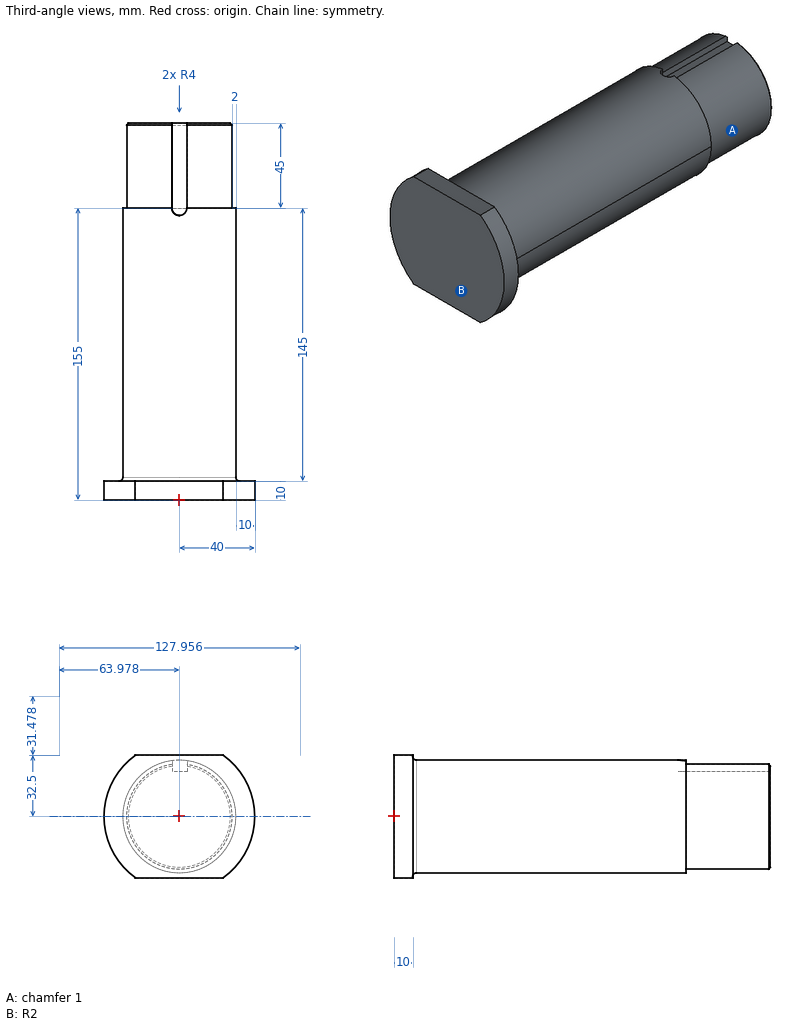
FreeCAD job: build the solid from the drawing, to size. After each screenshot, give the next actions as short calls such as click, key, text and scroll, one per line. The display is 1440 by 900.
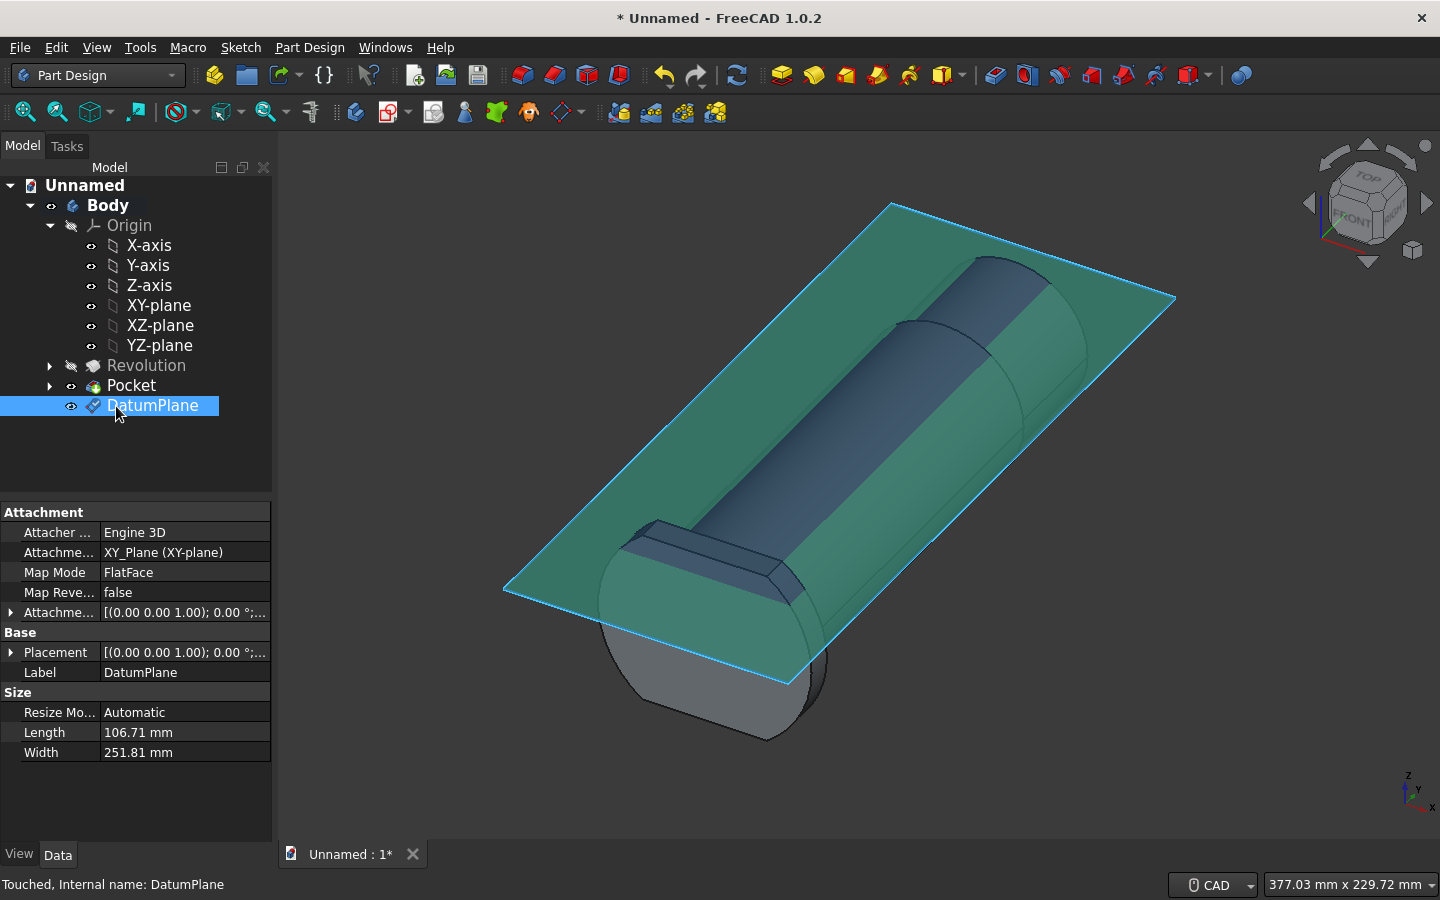
click(388, 112)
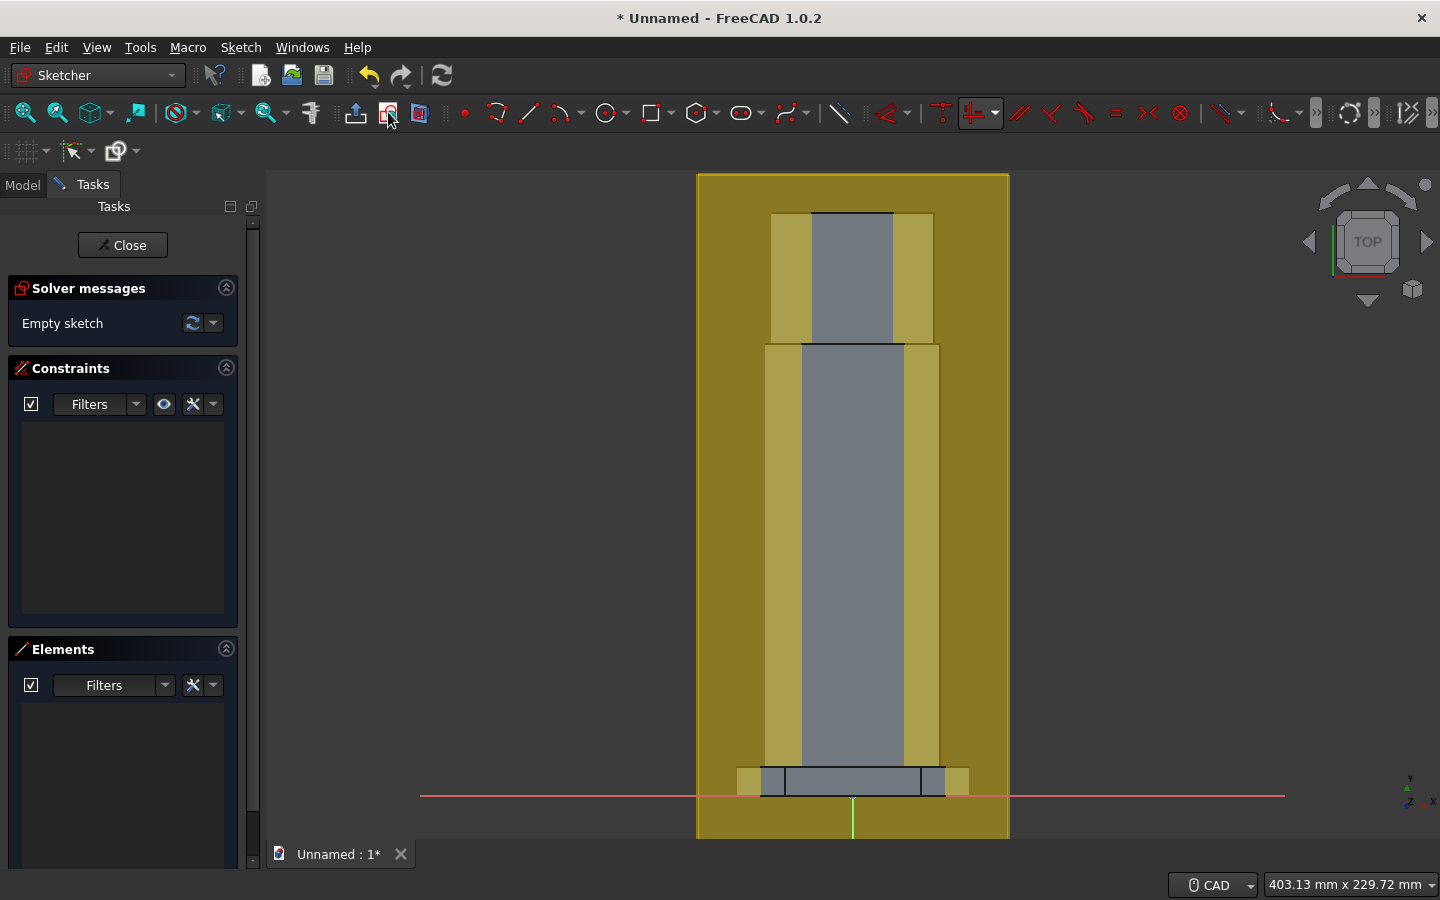
click(420, 114)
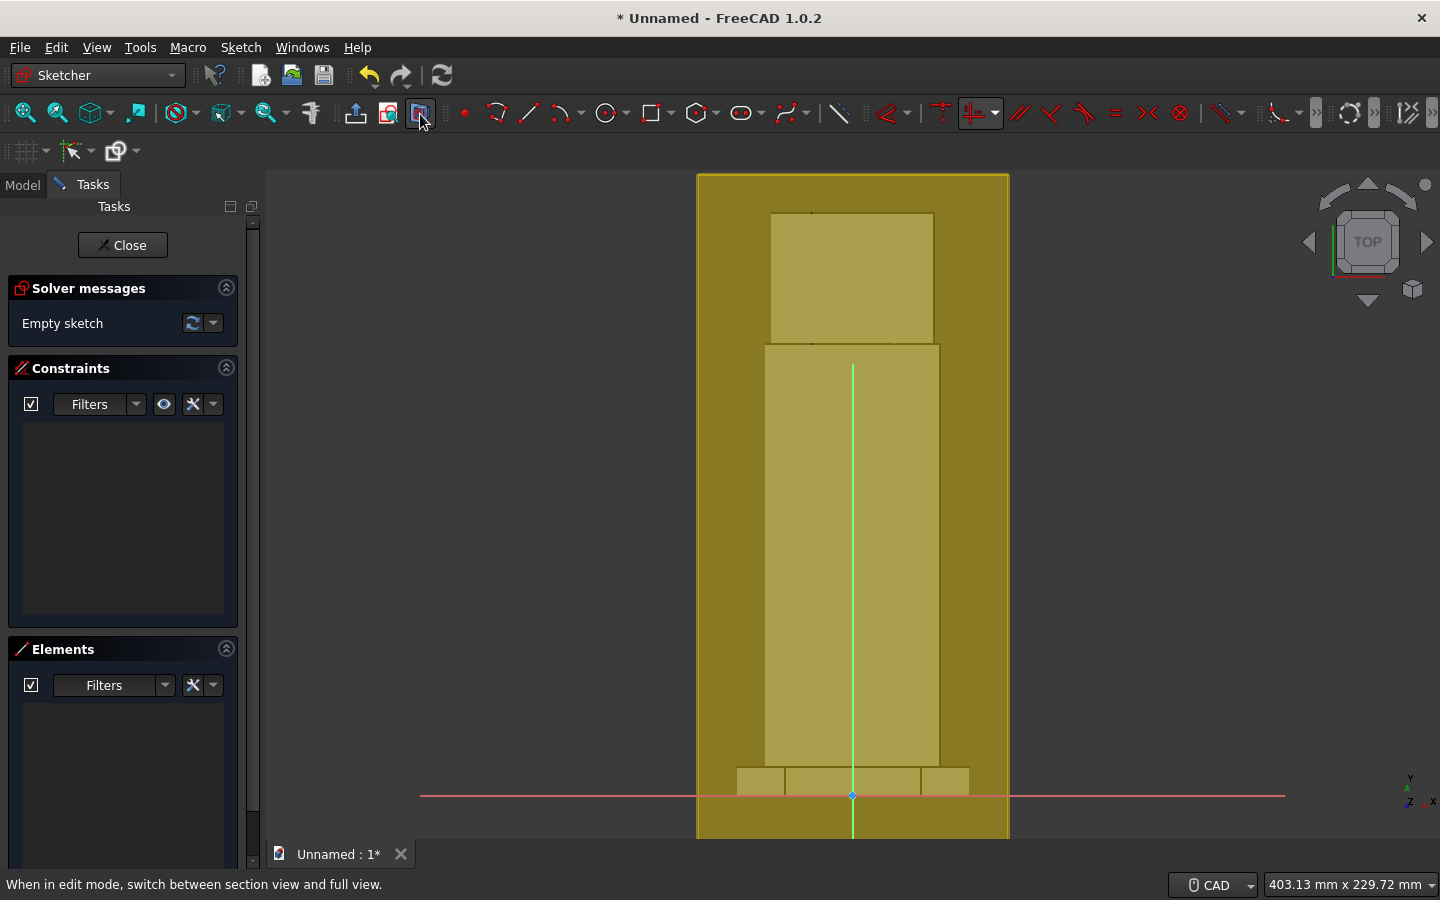
scroll(784, 504, down, 5)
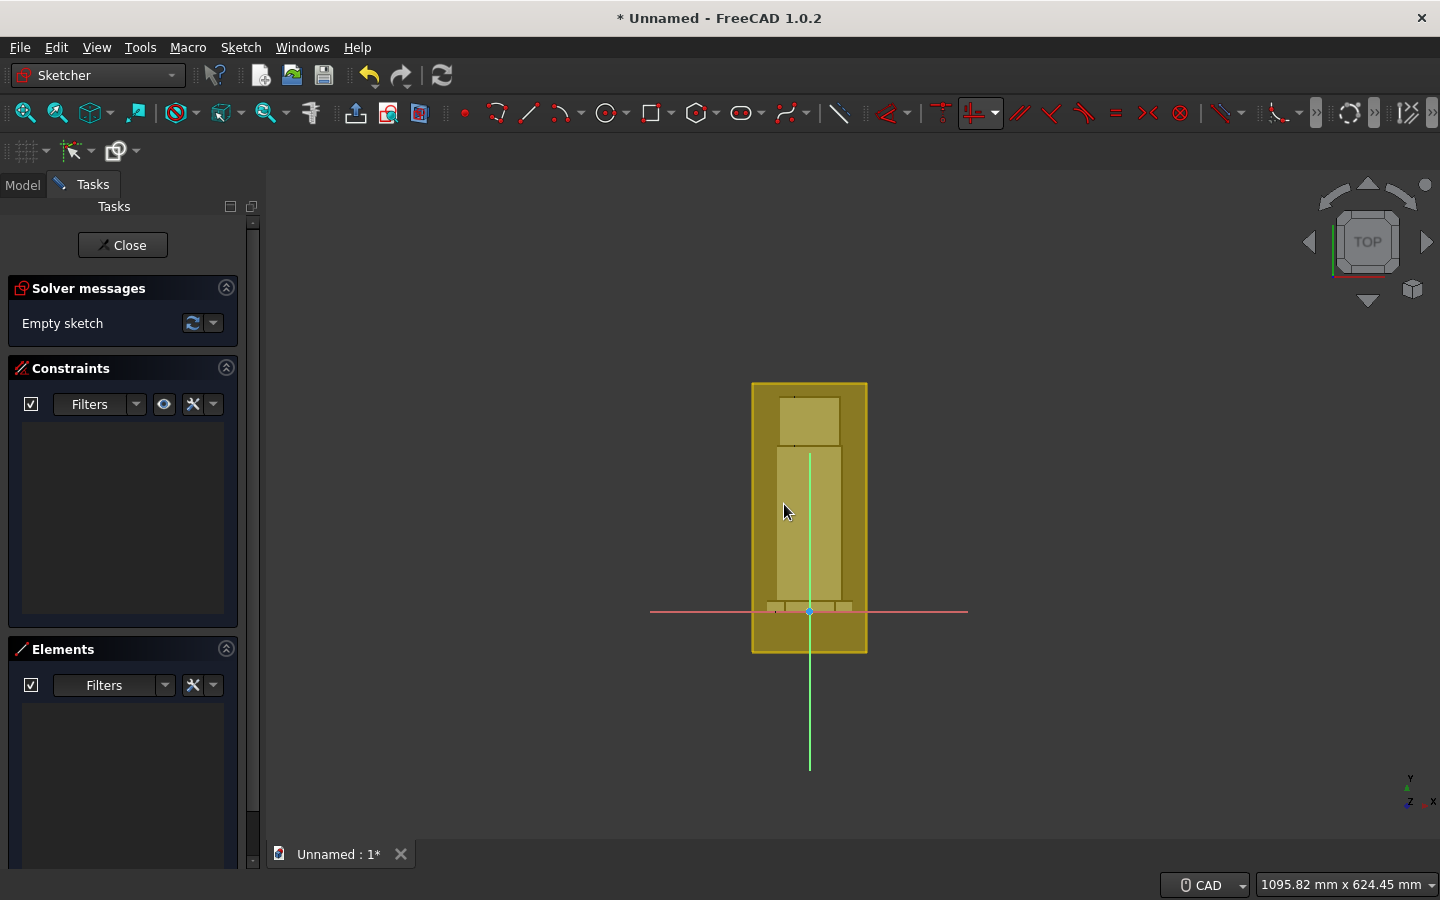
scroll(814, 408, up, 10)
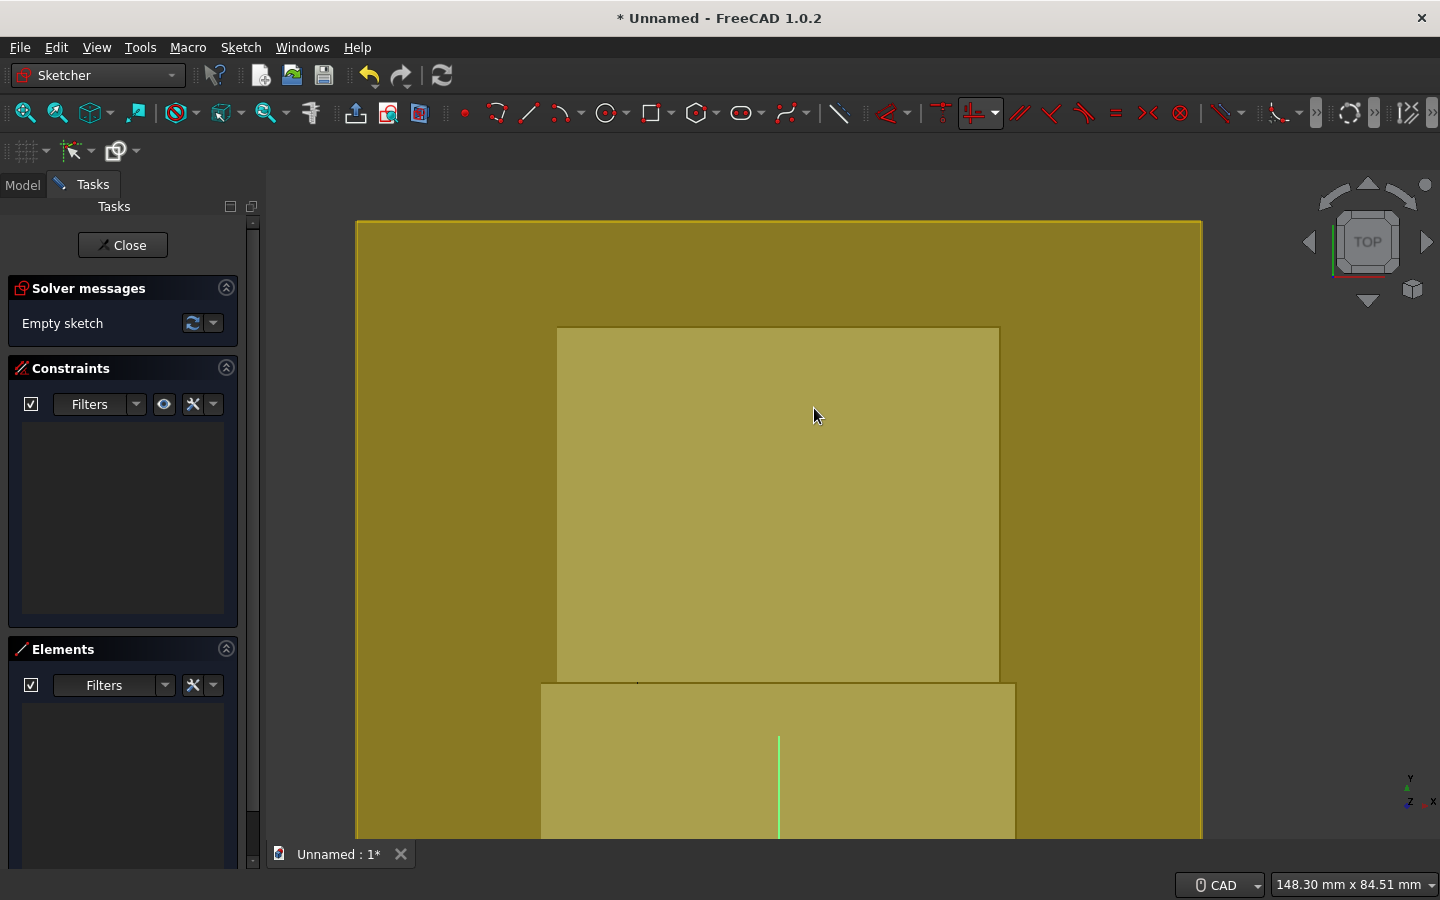
click(742, 114)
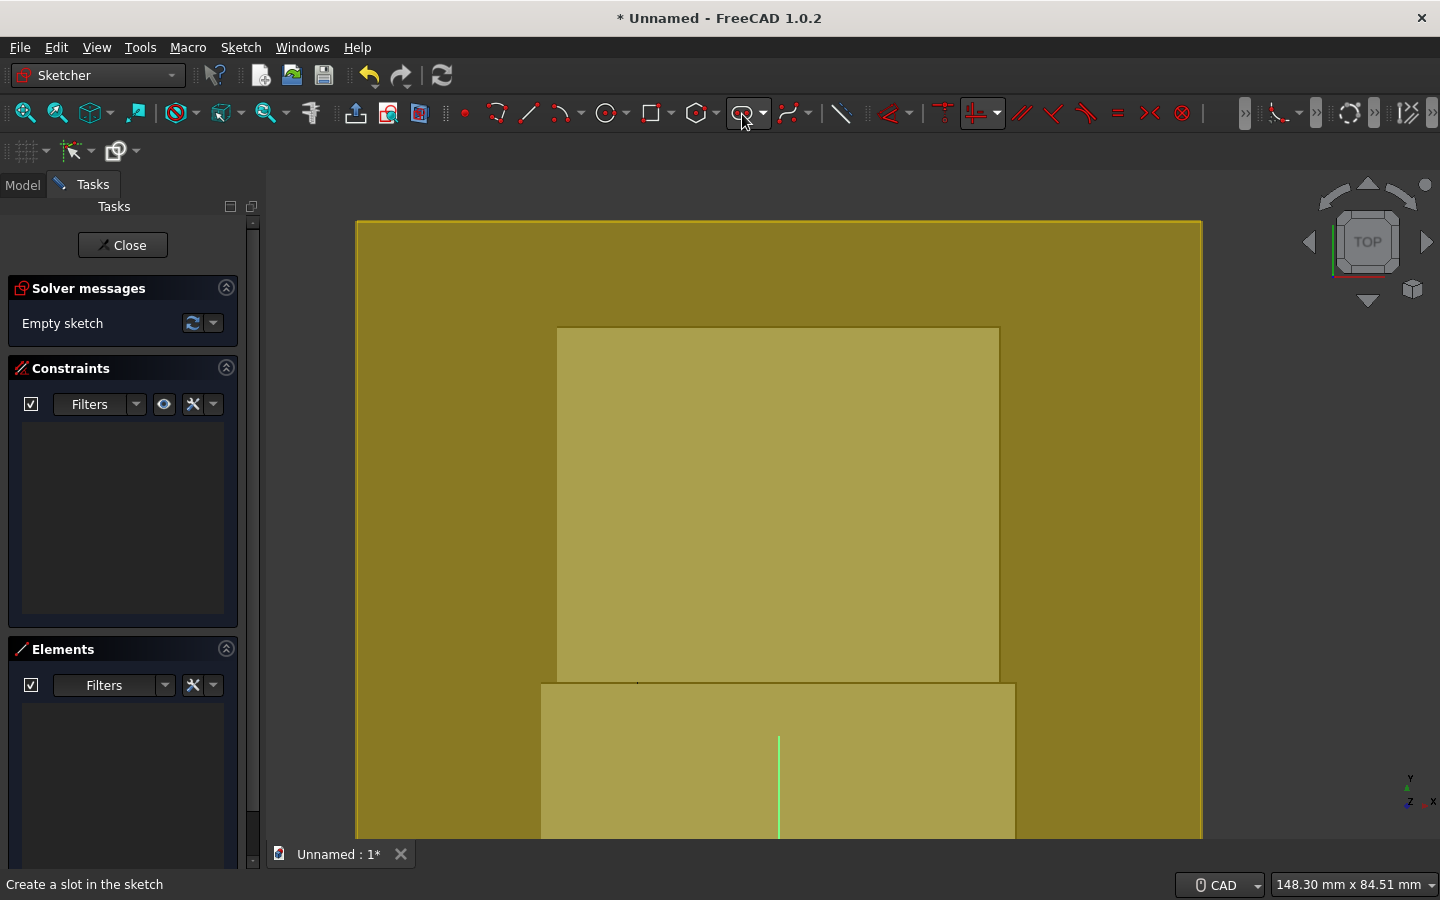
click(779, 683)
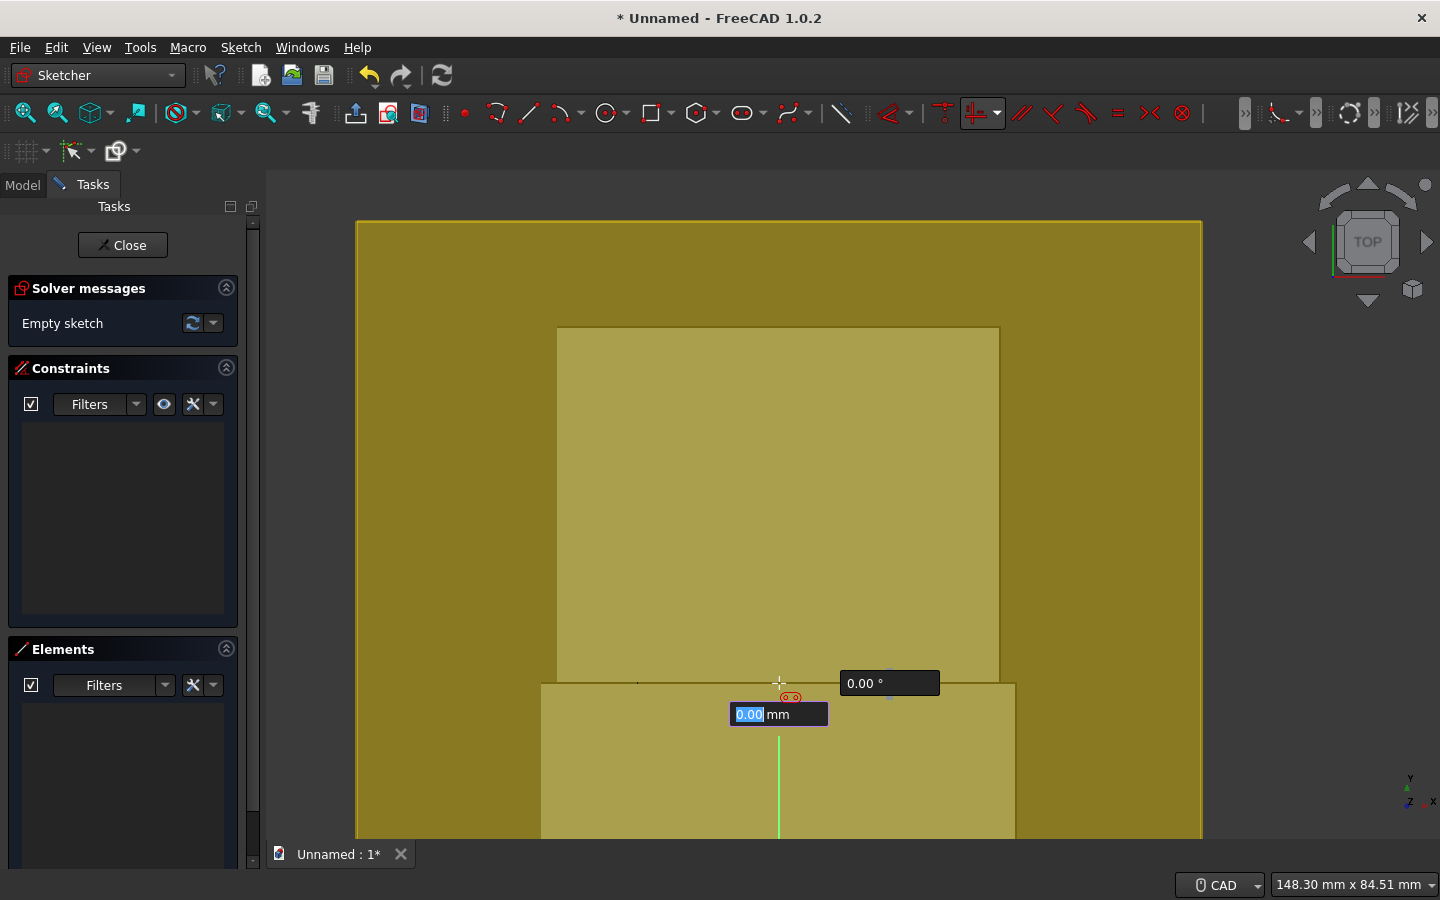
click(788, 327)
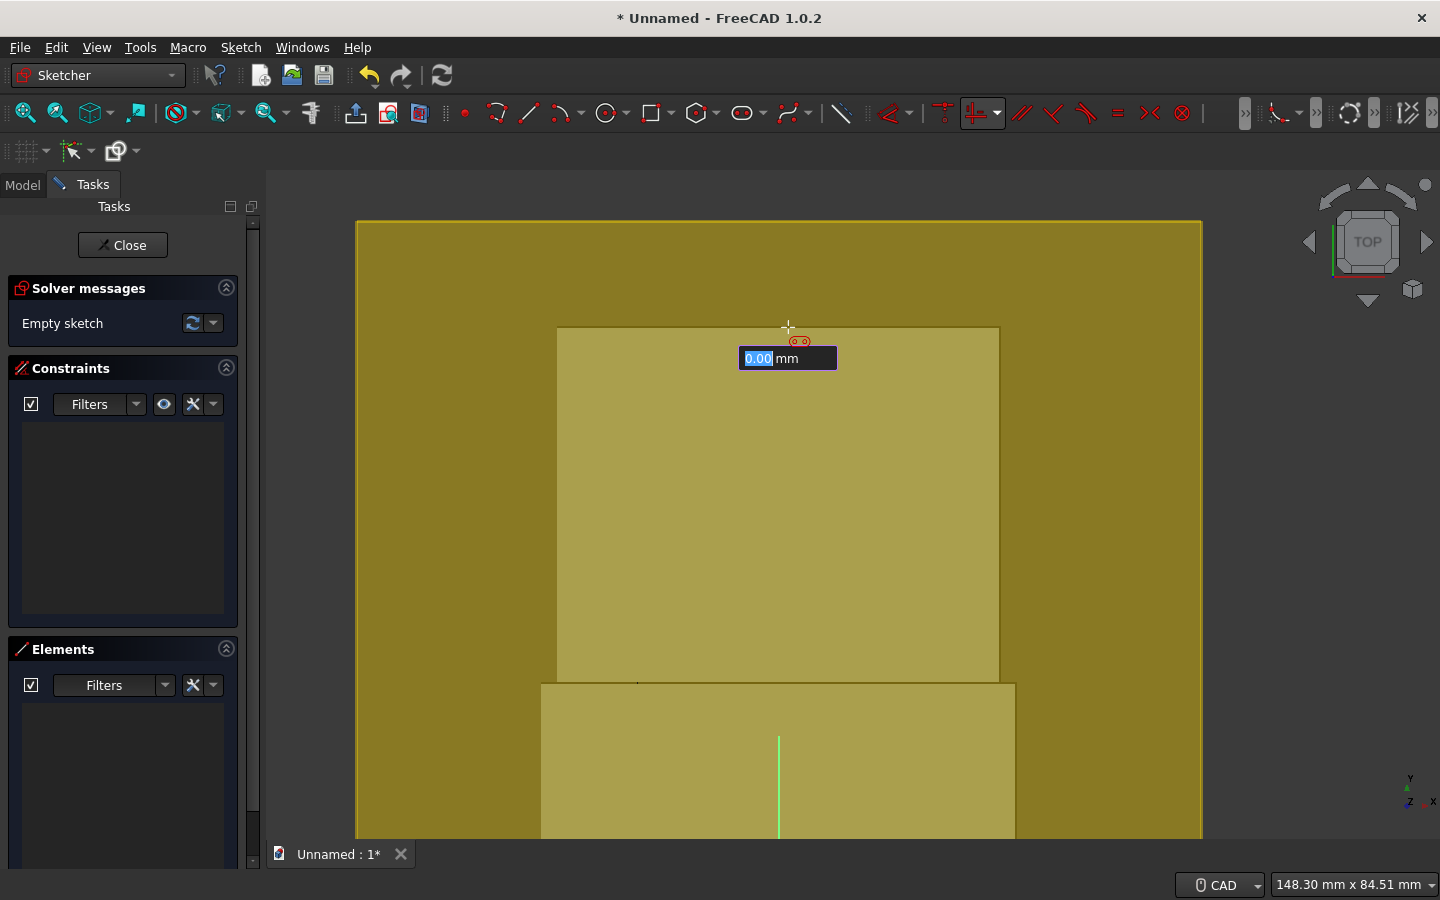
click(810, 505)
key(Escape)